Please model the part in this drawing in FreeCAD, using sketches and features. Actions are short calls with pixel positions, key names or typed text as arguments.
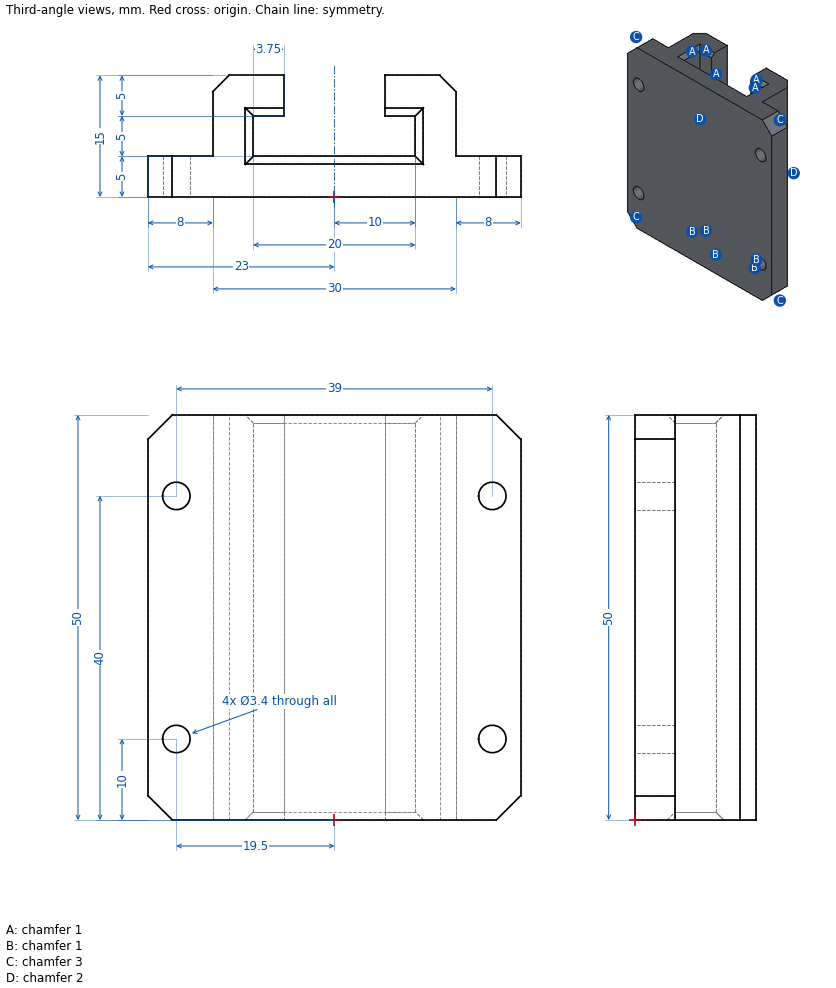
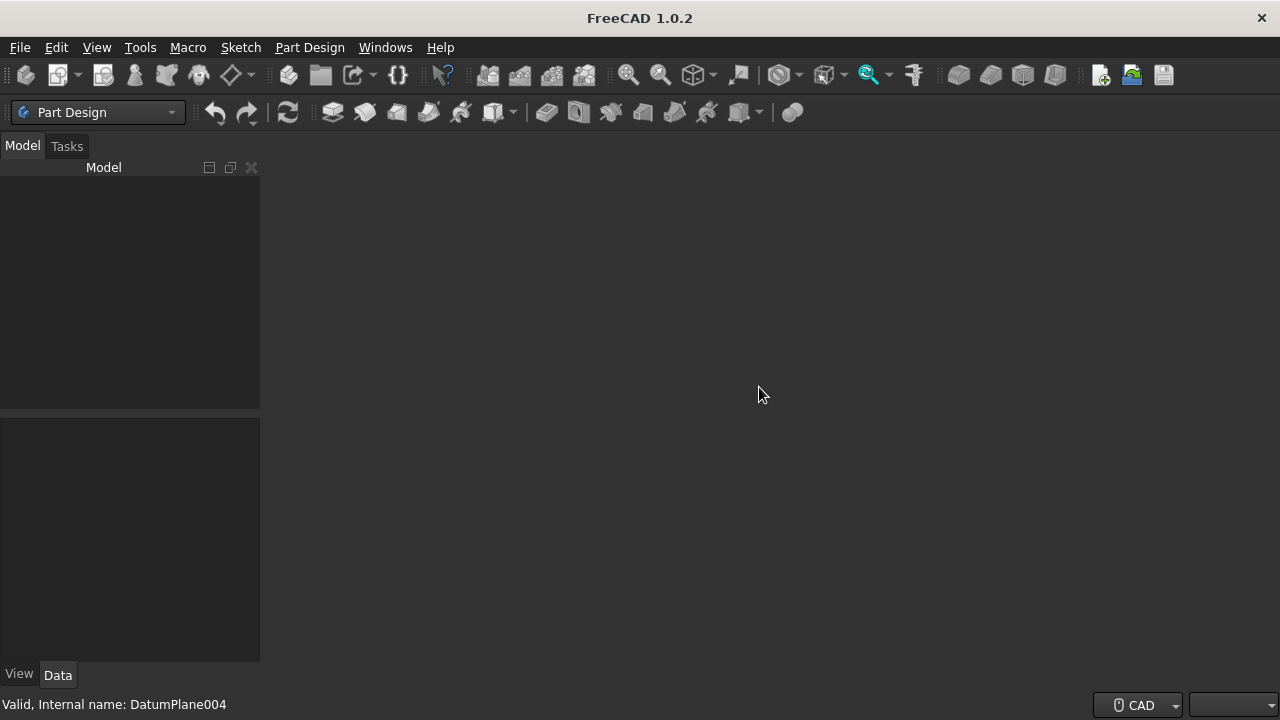
key(ctrl+n)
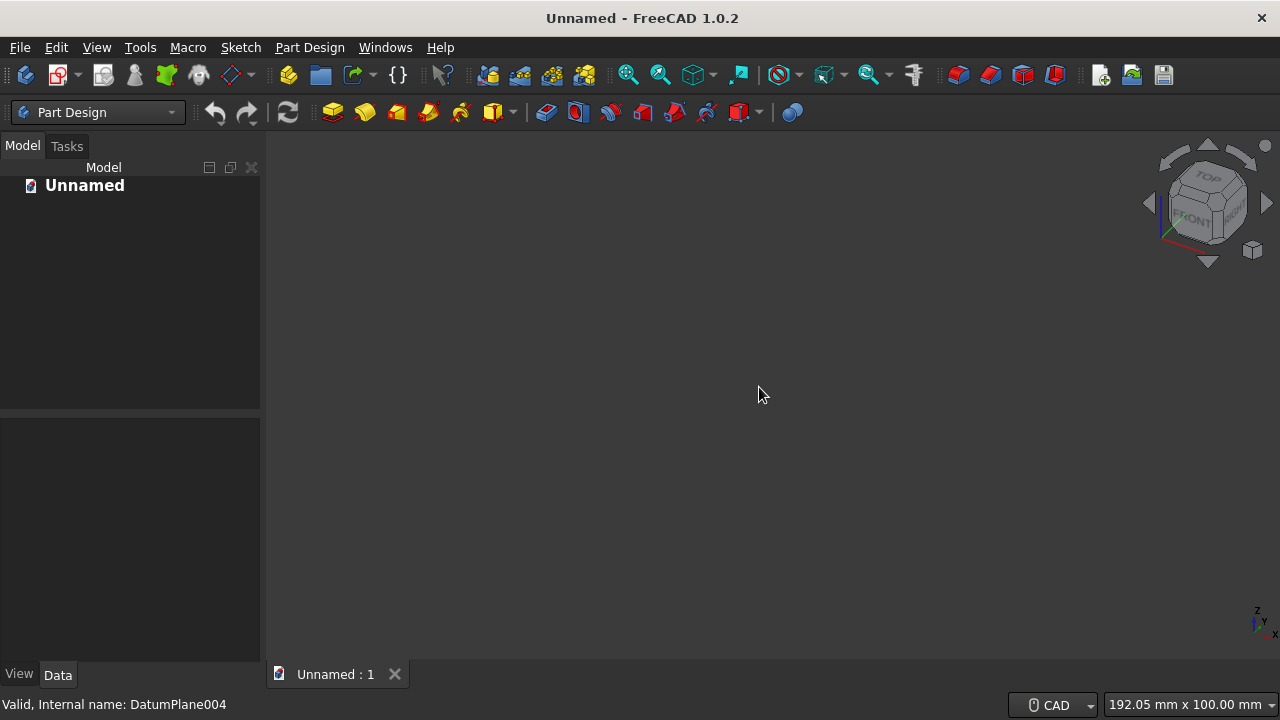
click(58, 76)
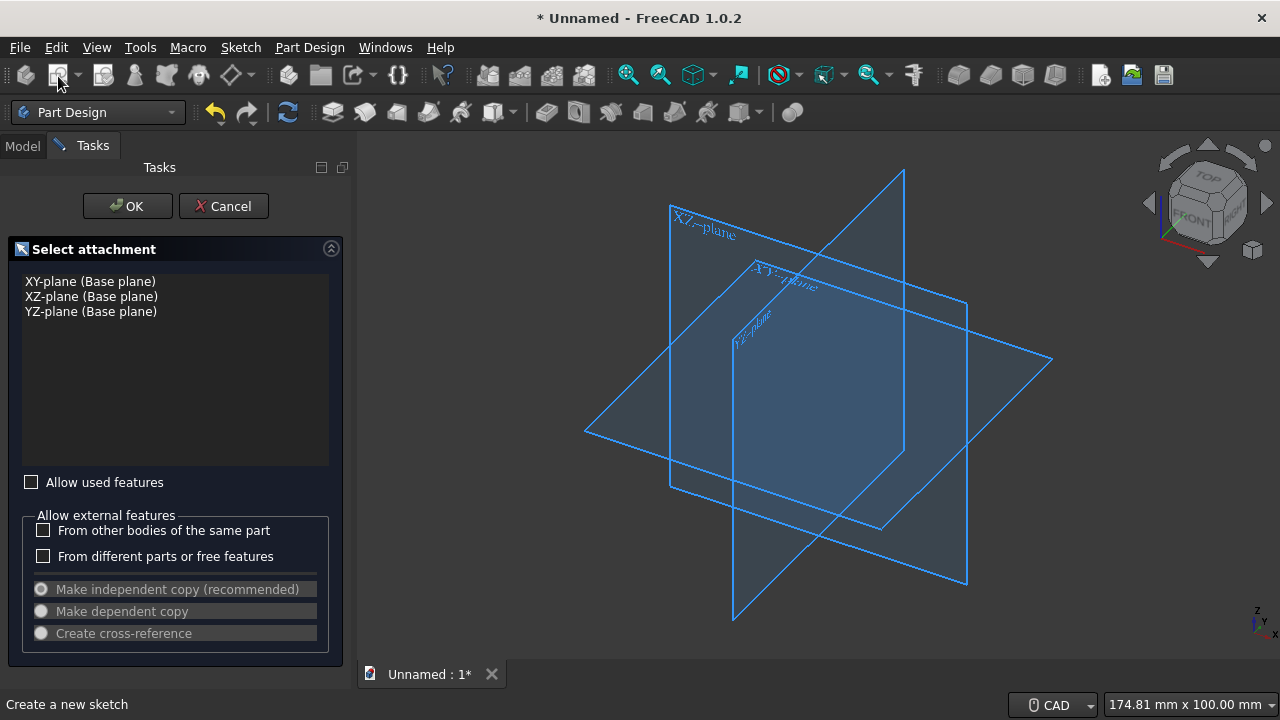
click(82, 282)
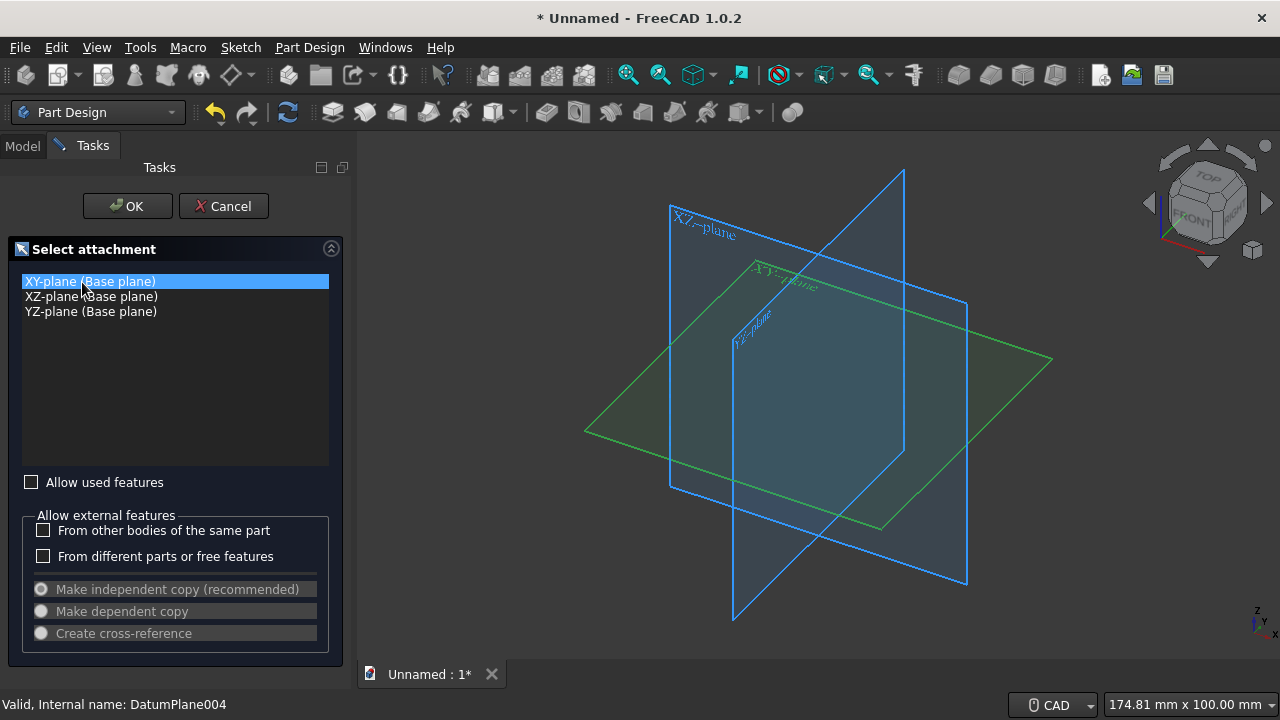
click(128, 206)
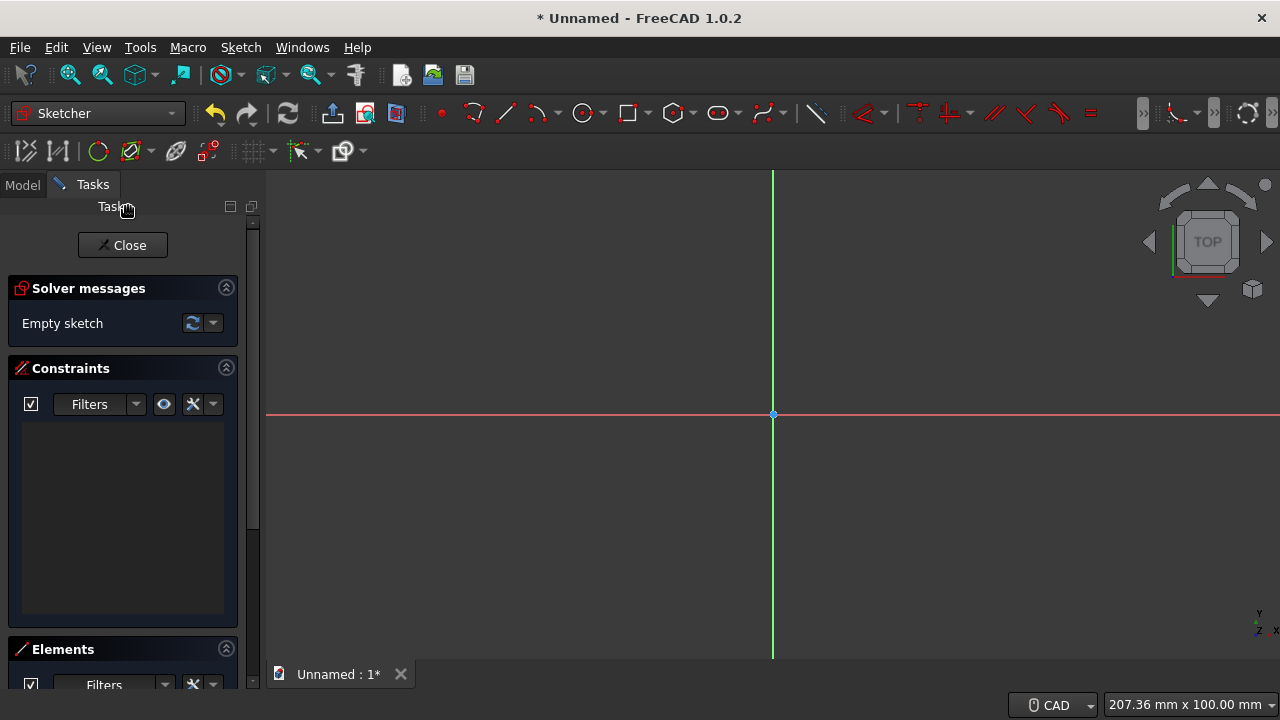
scroll(795, 366, up, 7)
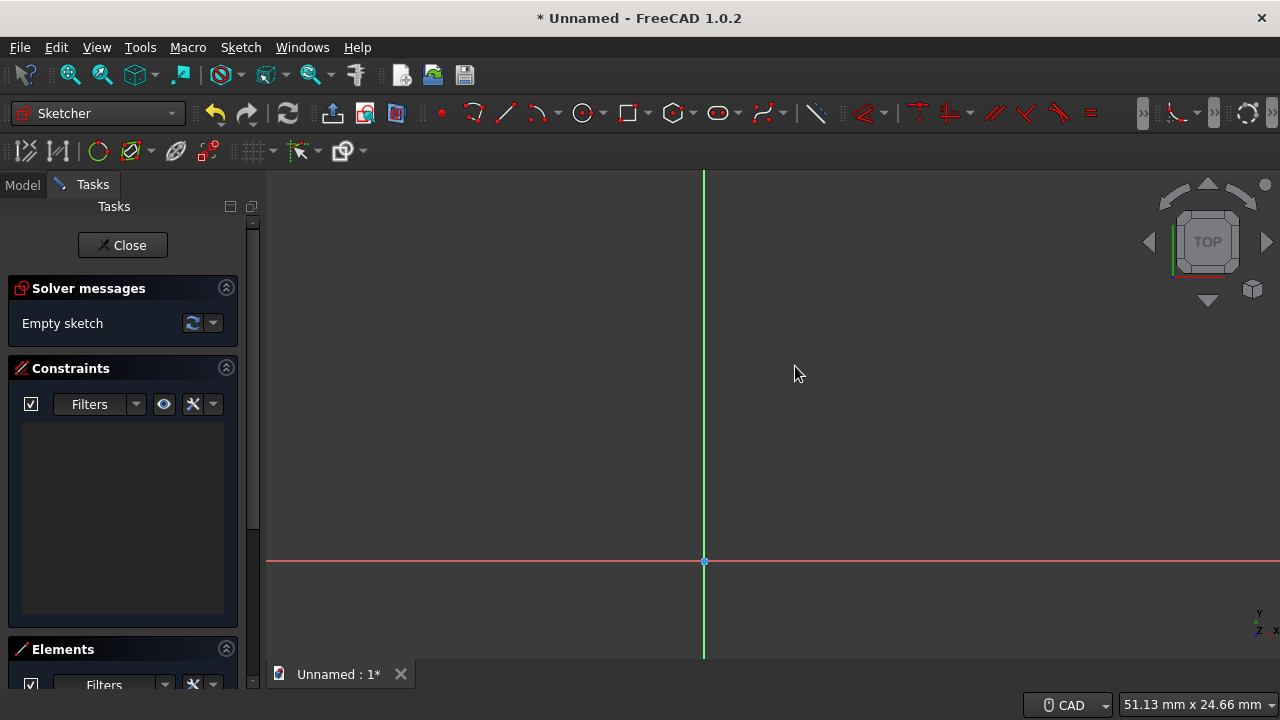
key(g)
key(m)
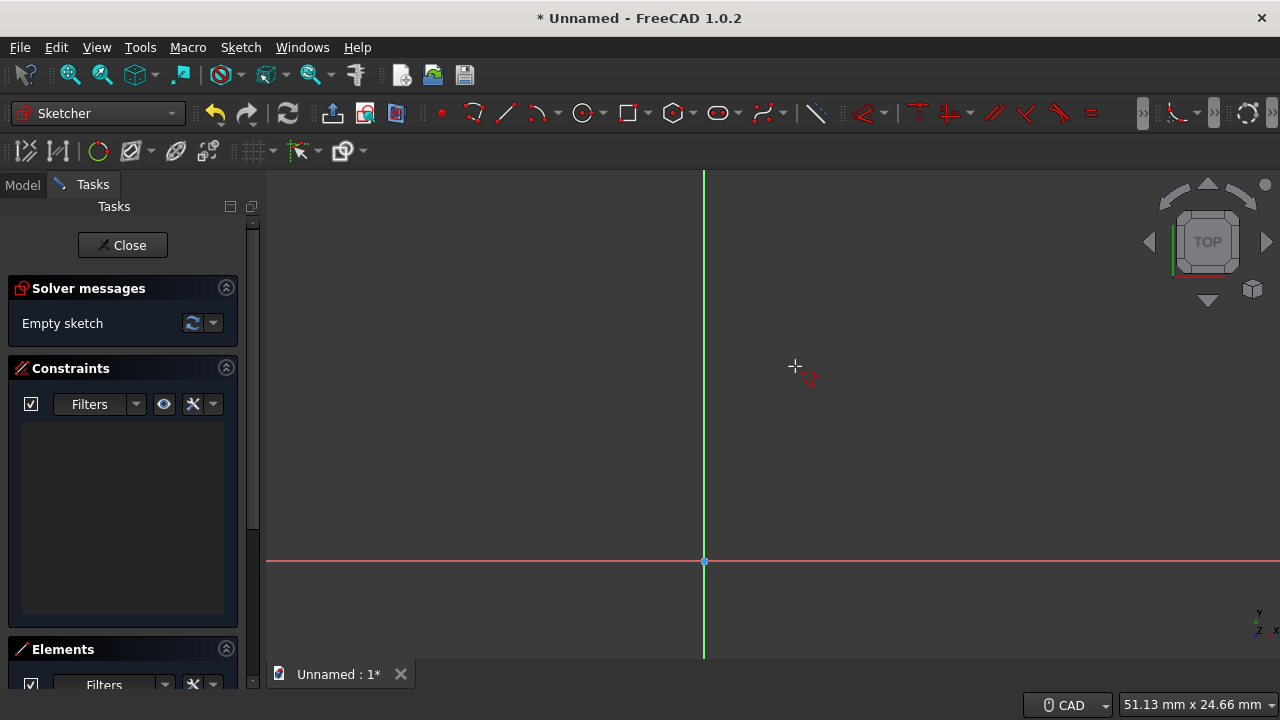
click(902, 462)
click(506, 462)
click(506, 363)
click(580, 363)
click(580, 264)
click(407, 264)
click(407, 561)
click(1002, 552)
click(1002, 264)
click(828, 264)
click(828, 363)
click(902, 363)
click(902, 463)
key(Escape)
key(Escape)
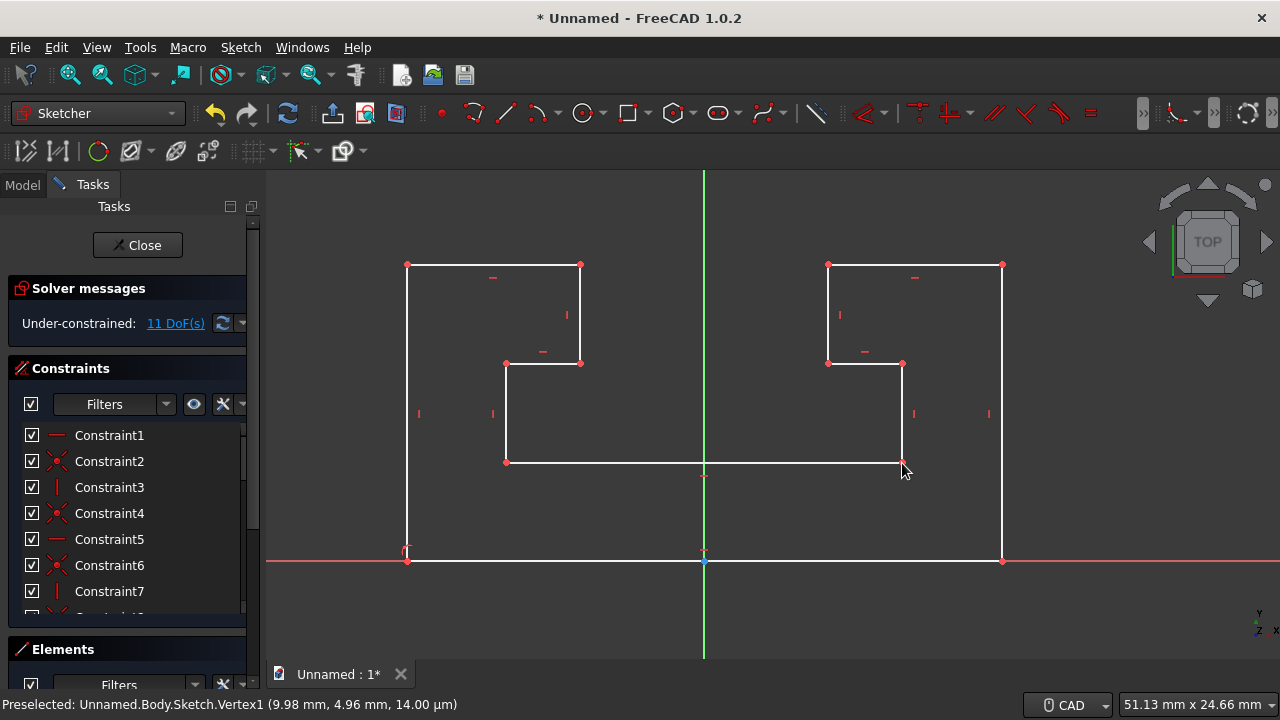
click(407, 265)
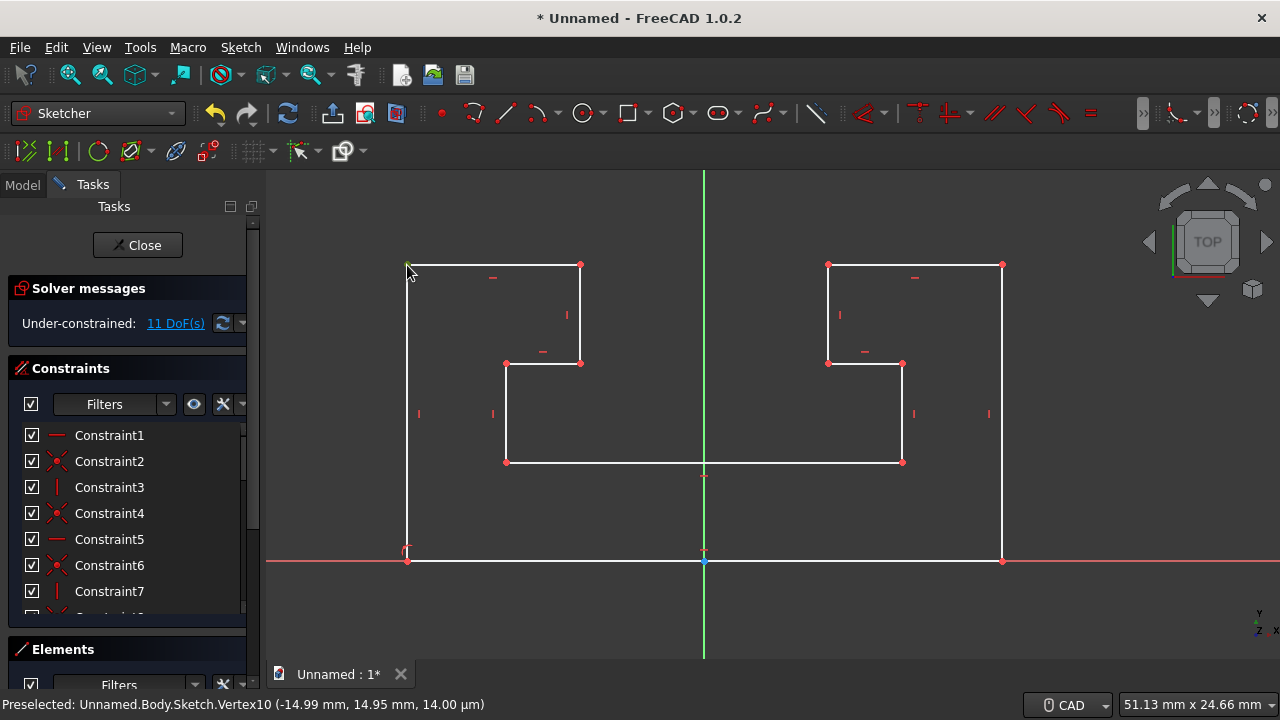
click(1002, 265)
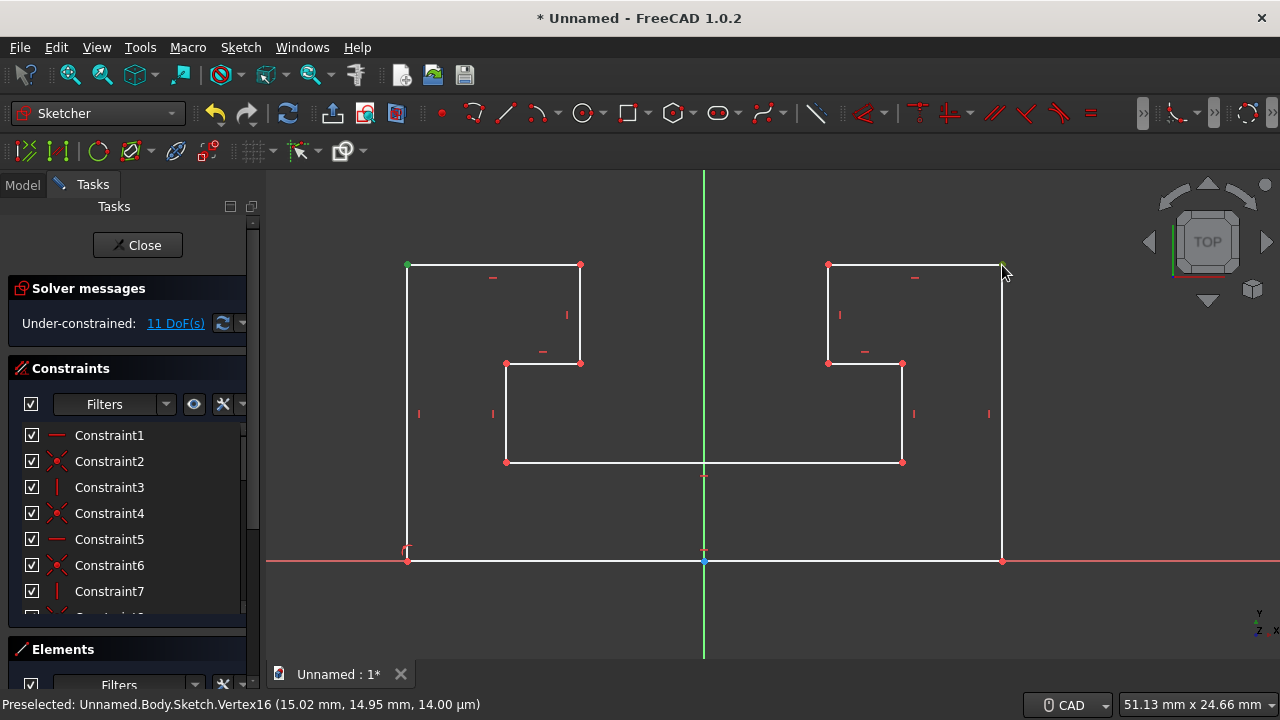
click(704, 600)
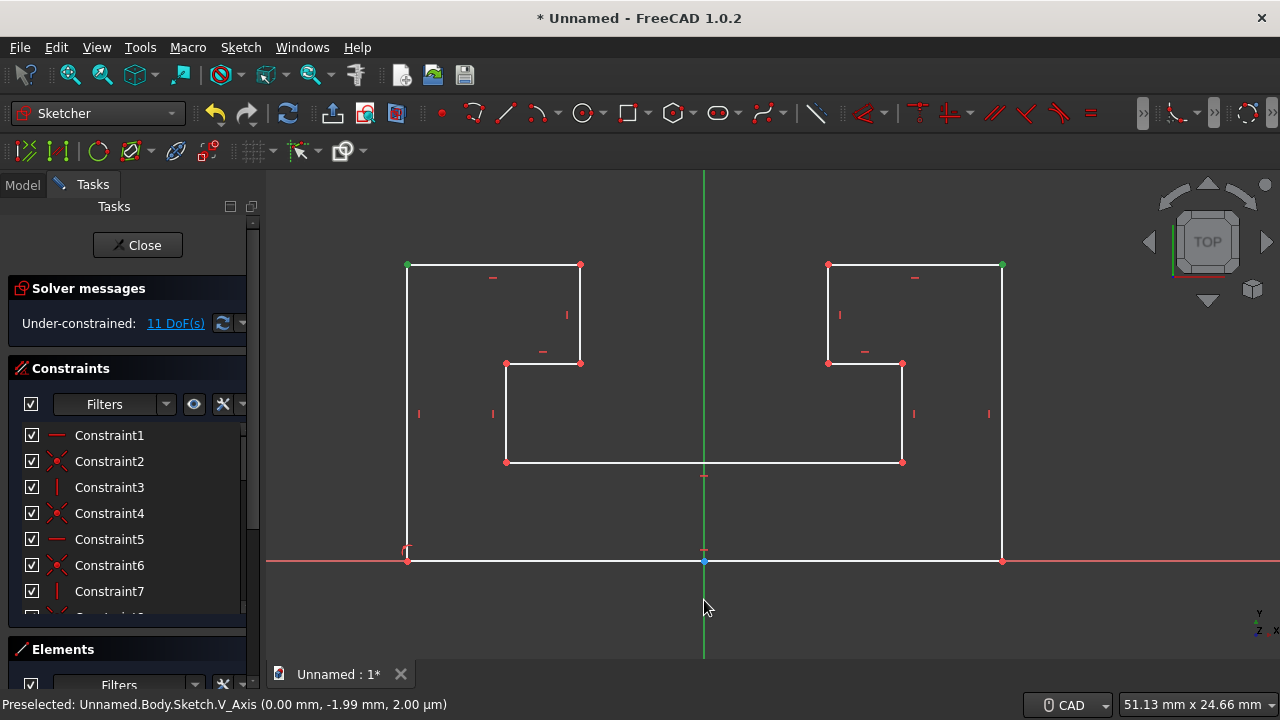
key(s)